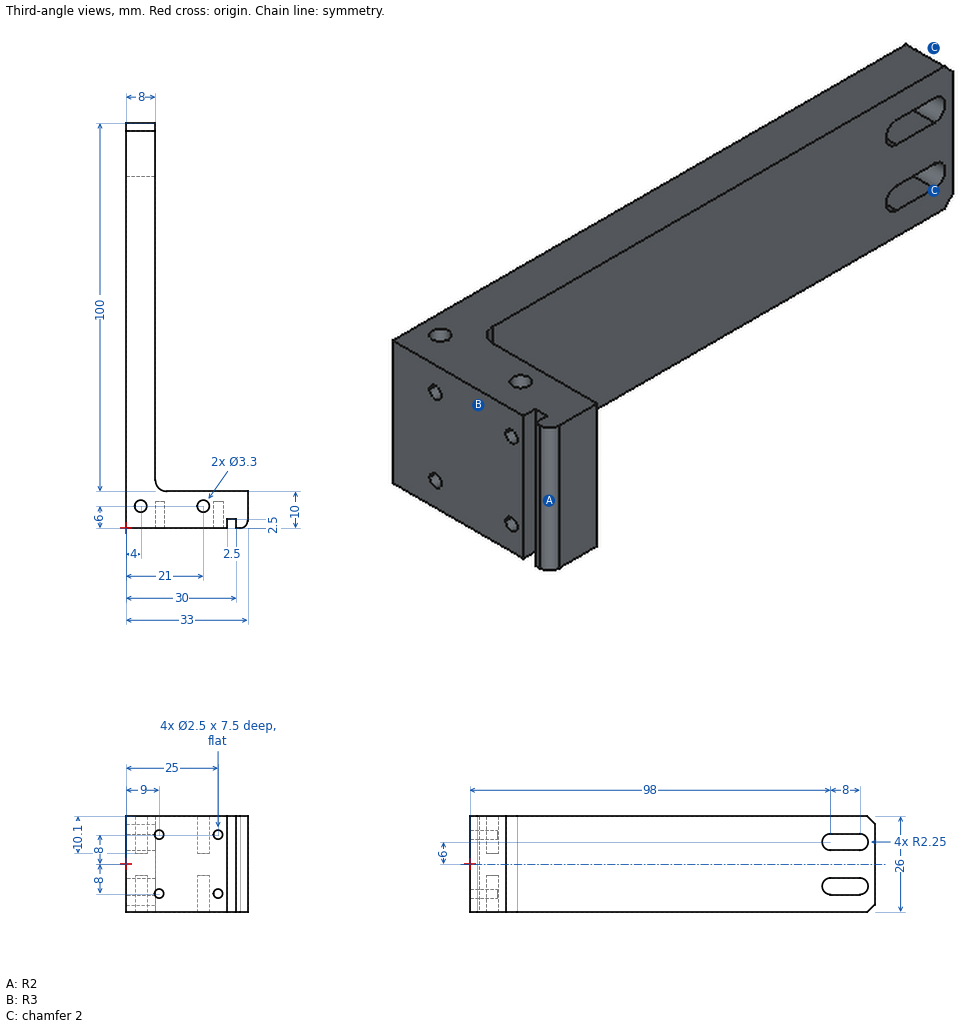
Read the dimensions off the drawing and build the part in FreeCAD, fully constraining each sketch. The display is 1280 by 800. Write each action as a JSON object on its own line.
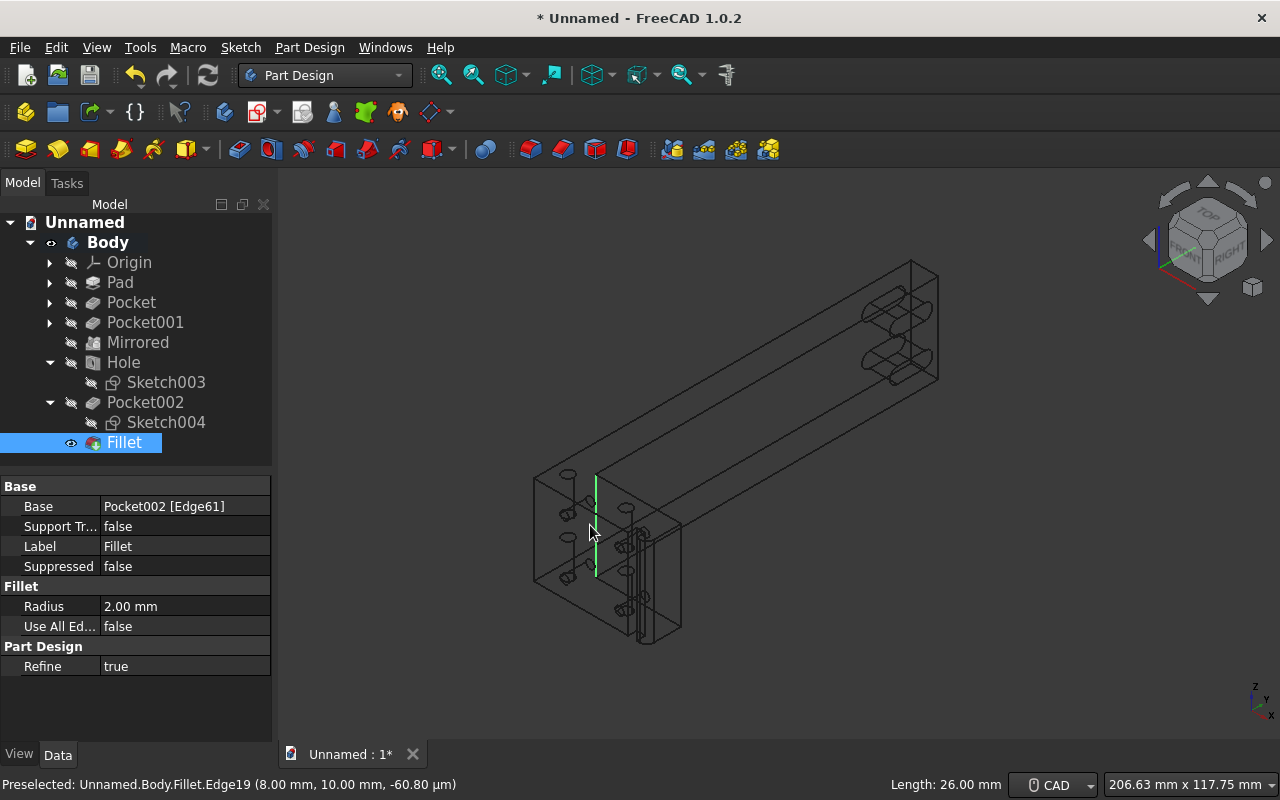
{"action": "key", "text": "v 1"}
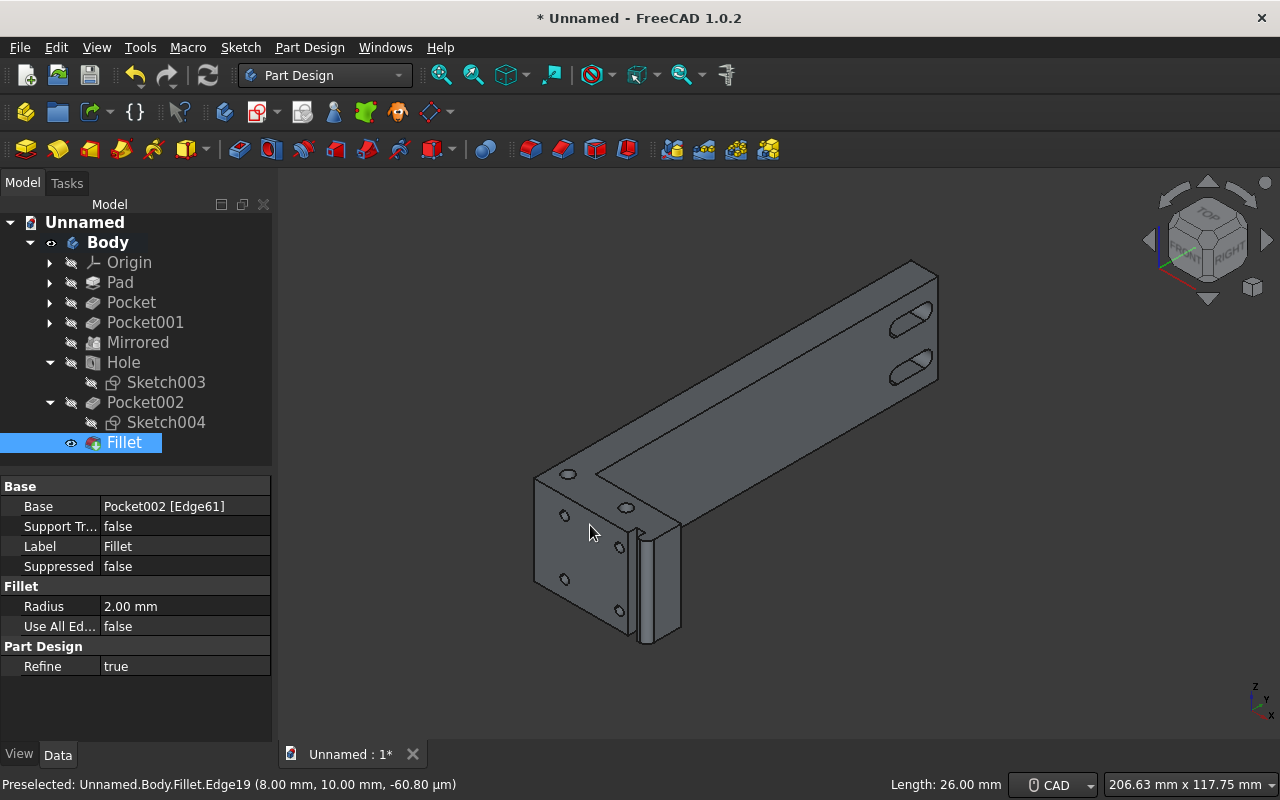
{"action": "left_click", "coordinate": [532, 150]}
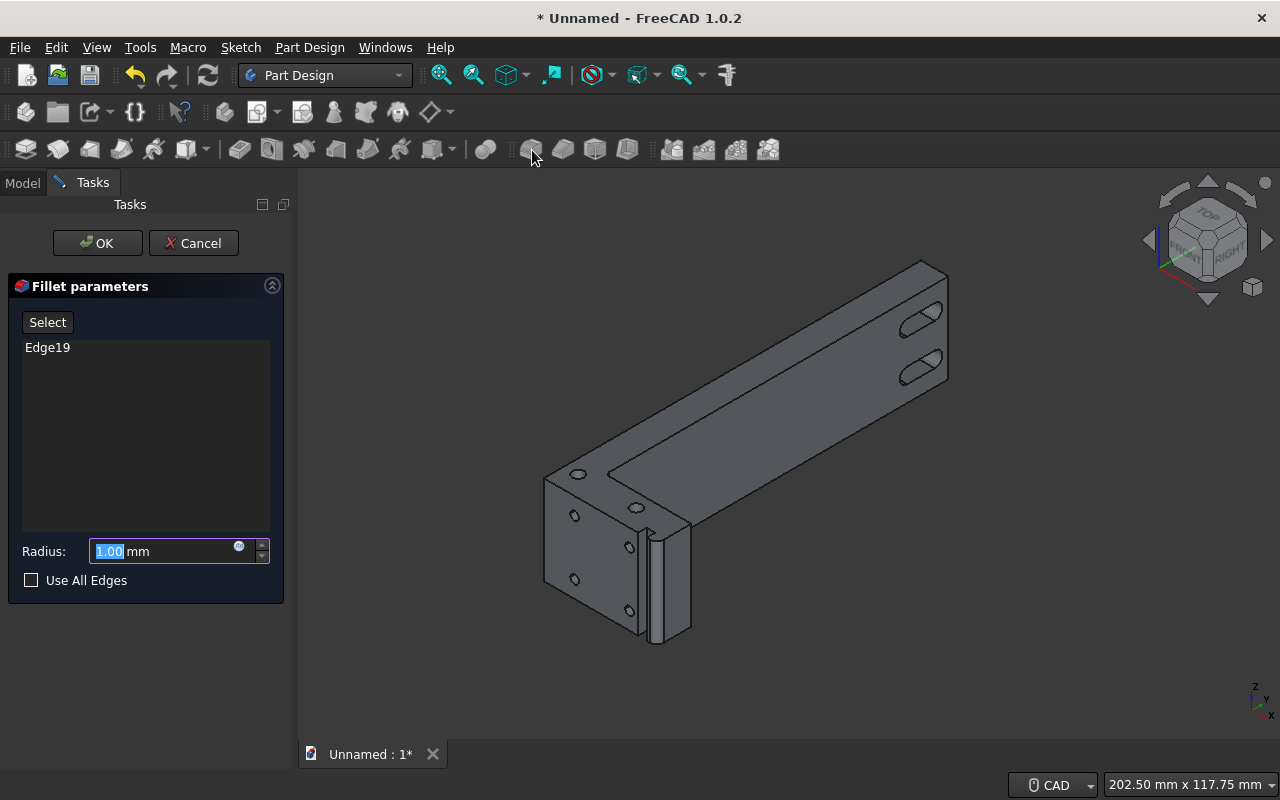
{"action": "type", "text": "3"}
{"action": "key", "text": "Tab"}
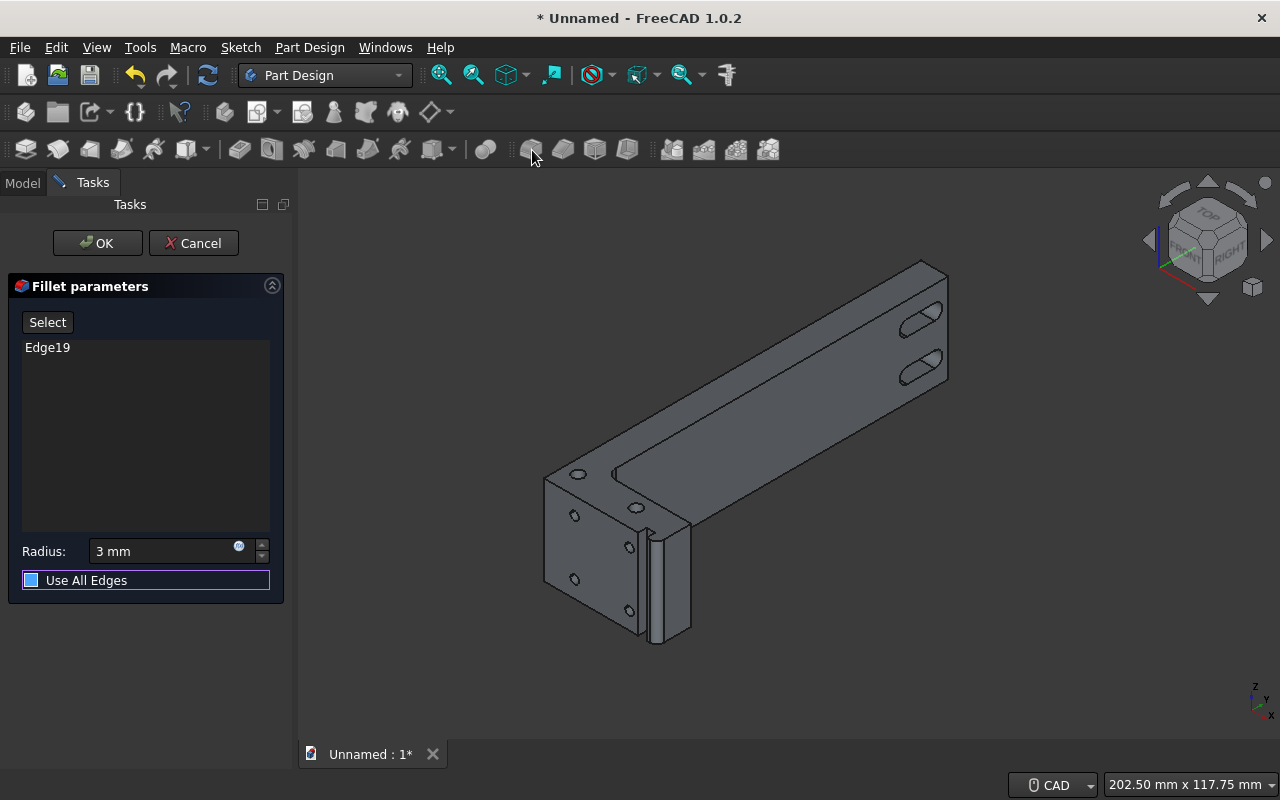
{"action": "left_click", "coordinate": [98, 243]}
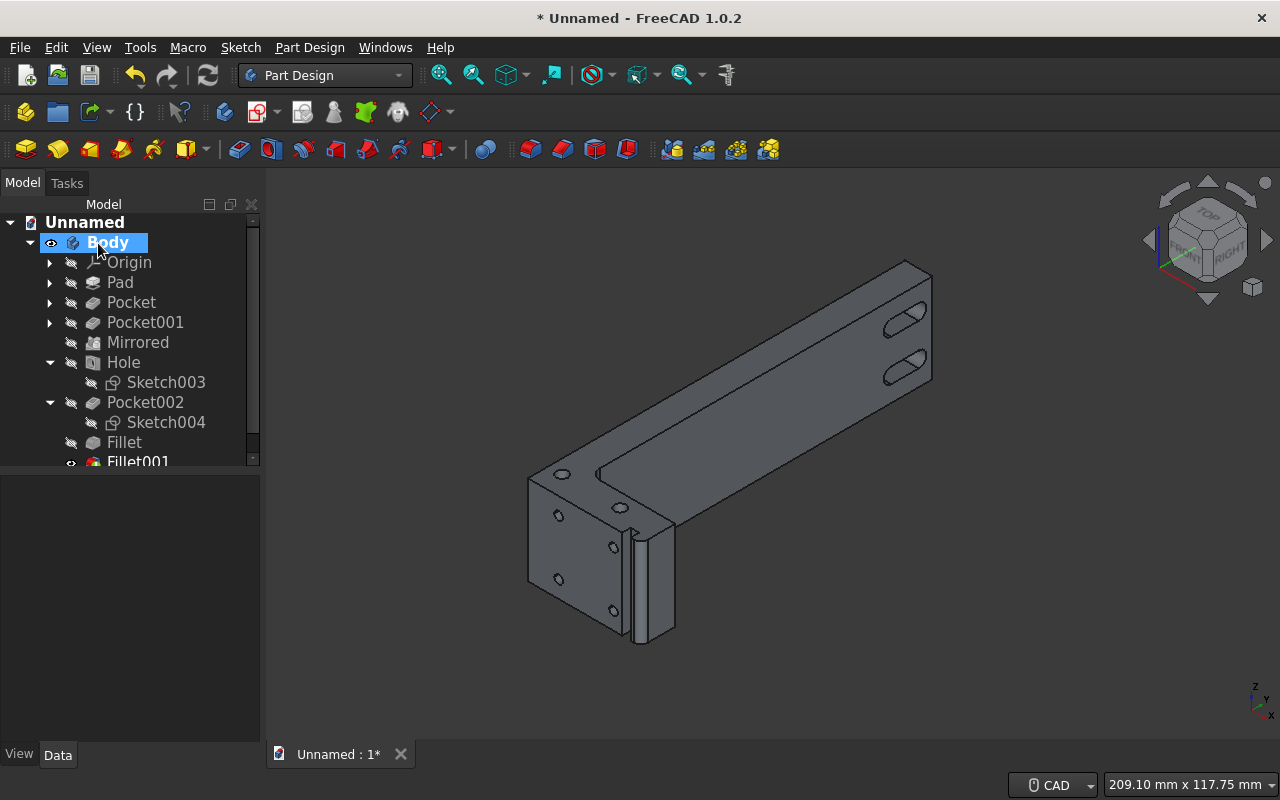
{"action": "key", "text": "2"}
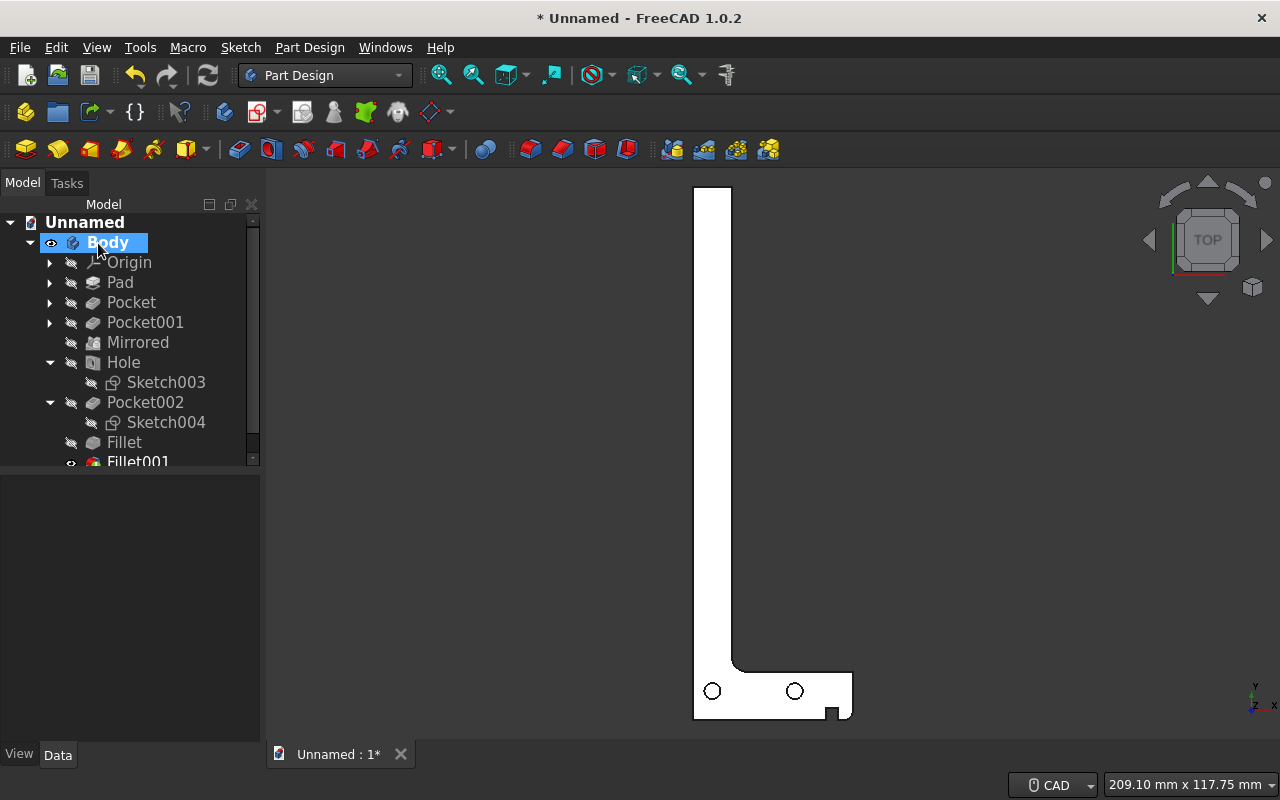
{"action": "key", "text": "0"}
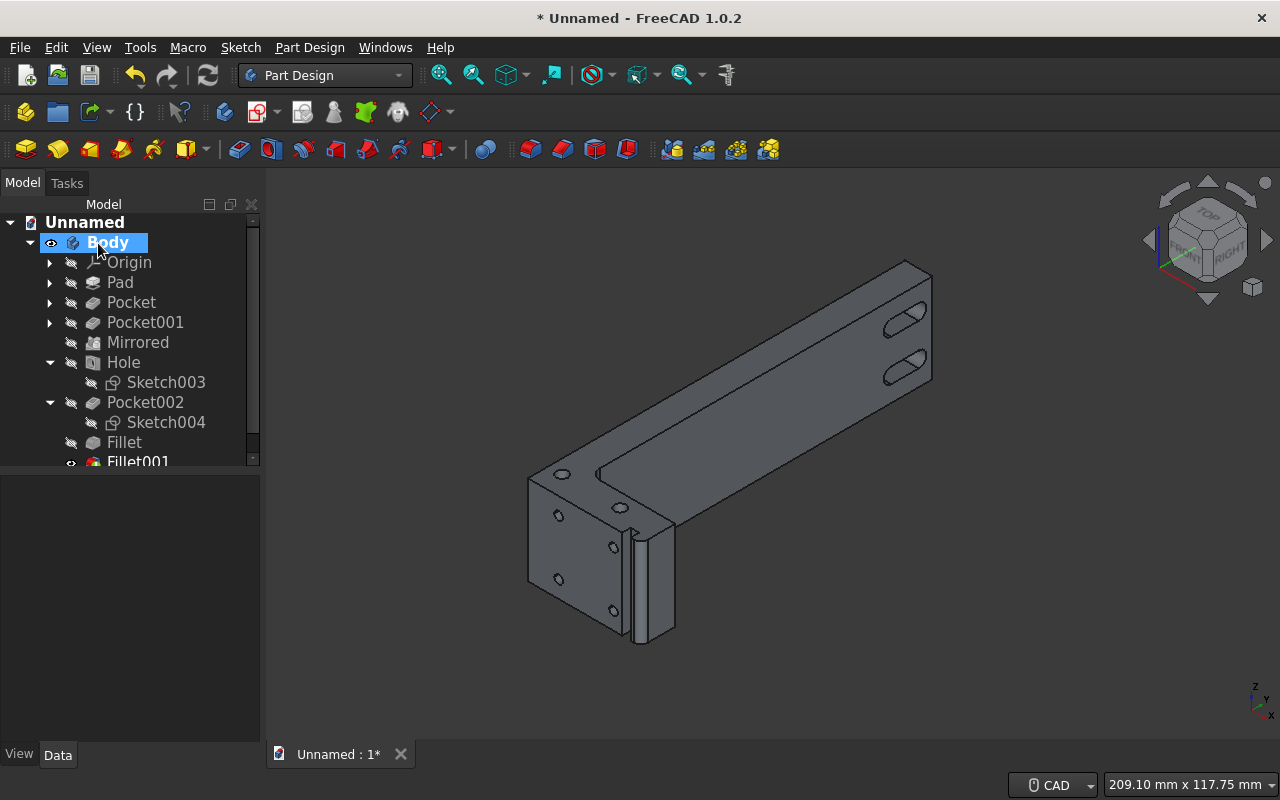
{"action": "key", "text": "1"}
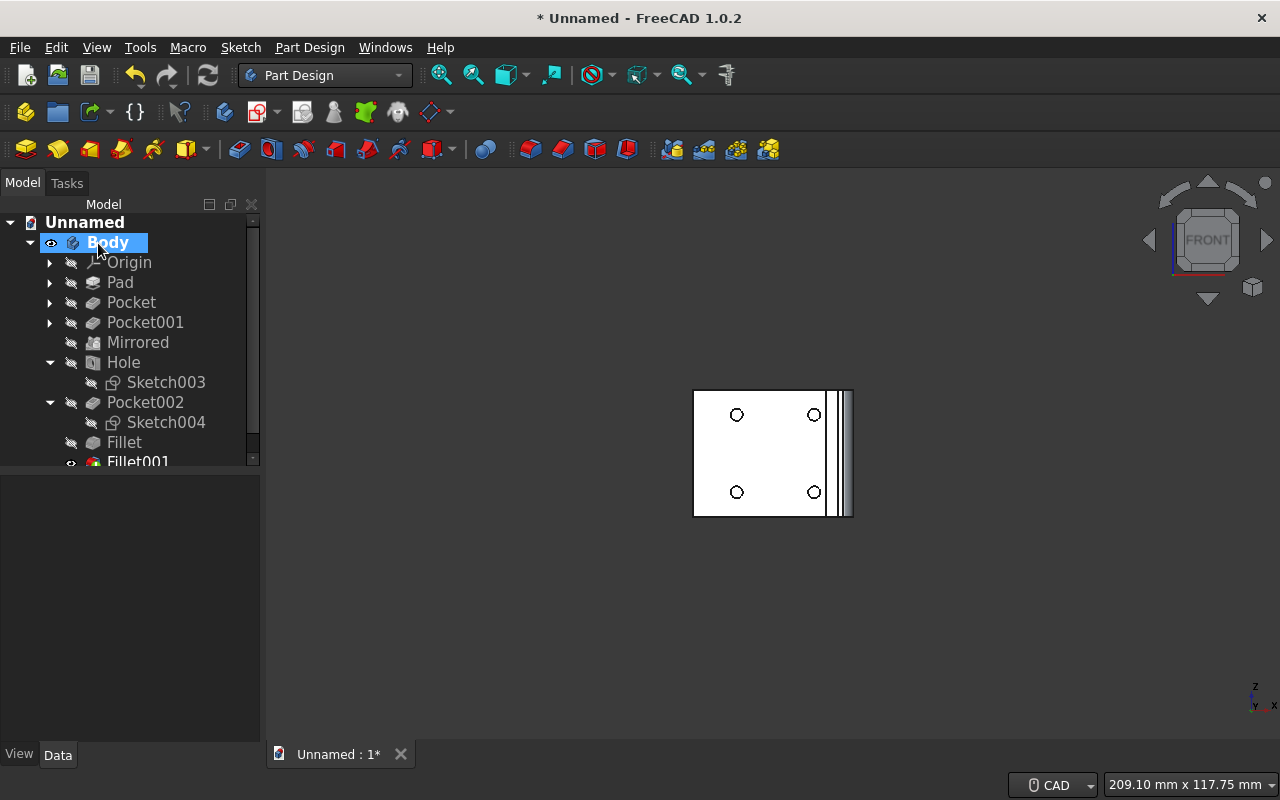
{"action": "left_click", "coordinate": [442, 76]}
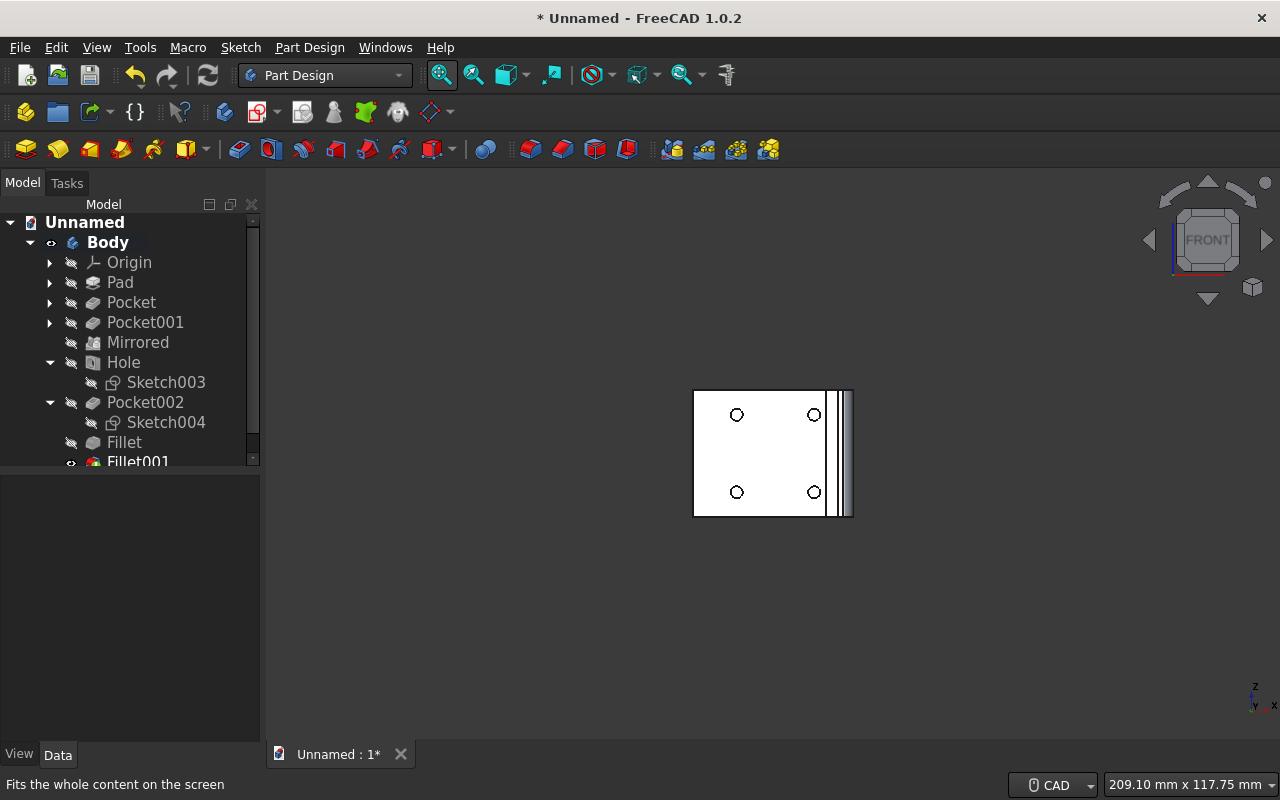
{"action": "key", "text": "3"}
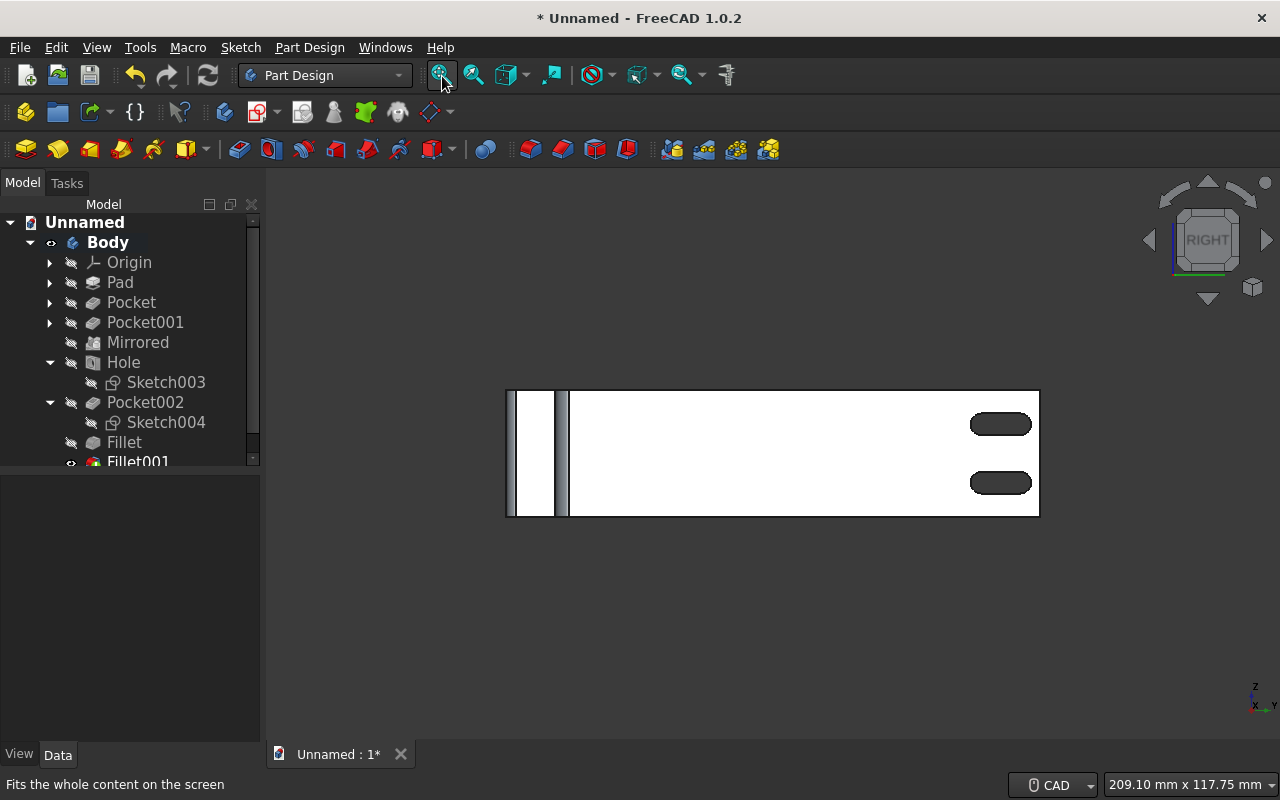
{"action": "key", "text": "5"}